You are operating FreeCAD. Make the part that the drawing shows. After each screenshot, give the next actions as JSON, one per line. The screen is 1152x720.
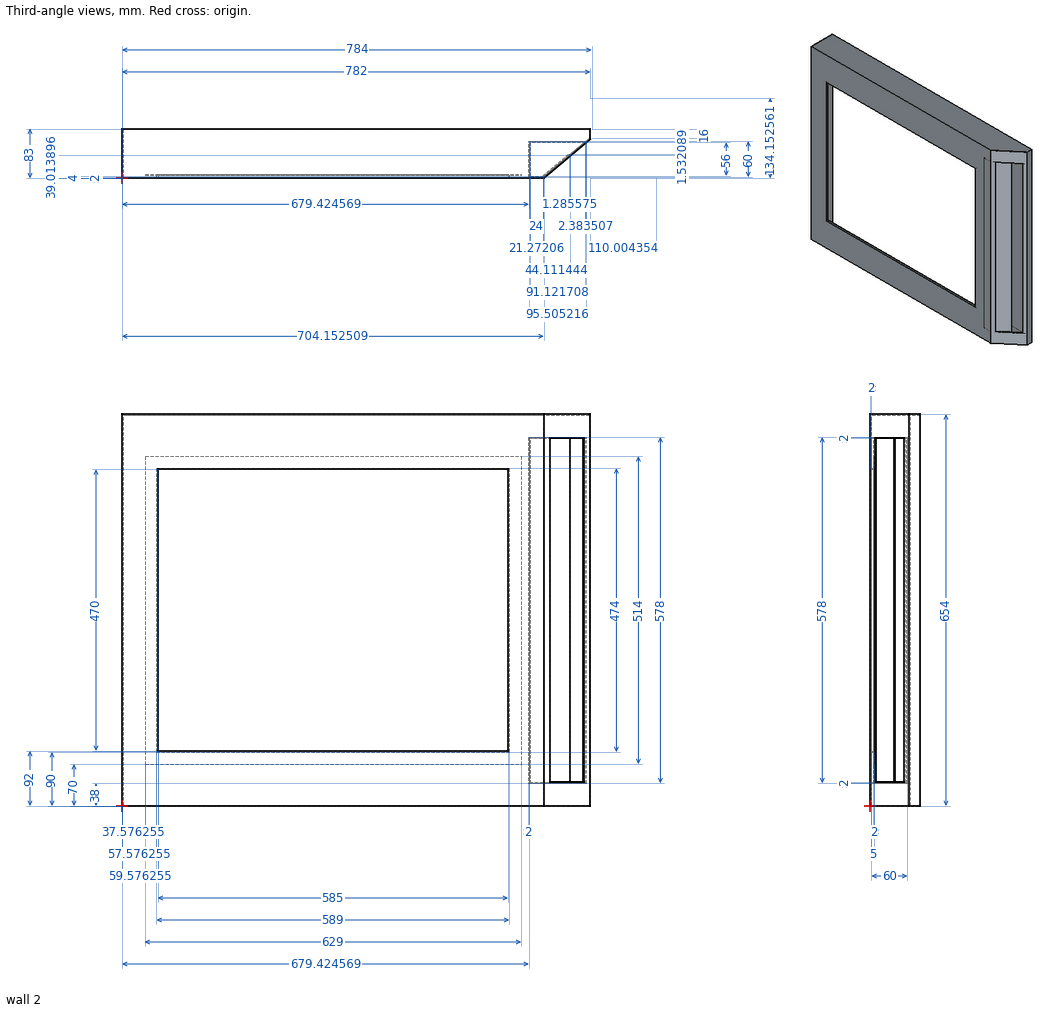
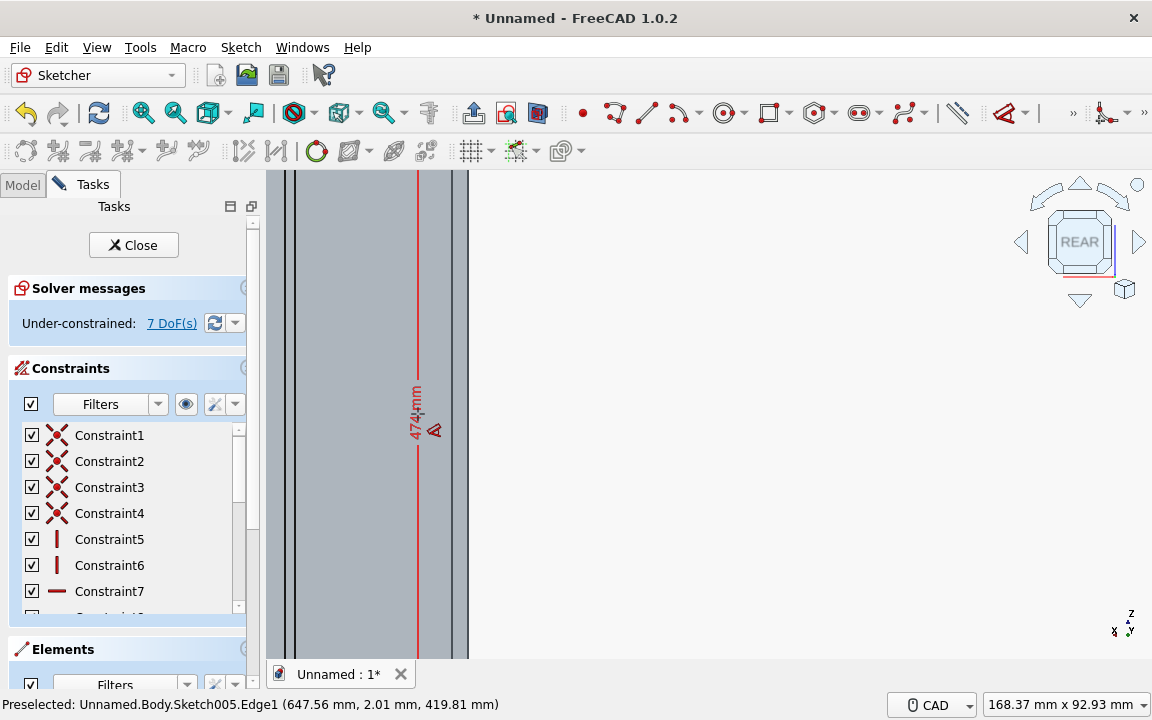
{"action": "scroll", "coordinate": [451, 334], "scroll_direction": "down", "scroll_amount": 11}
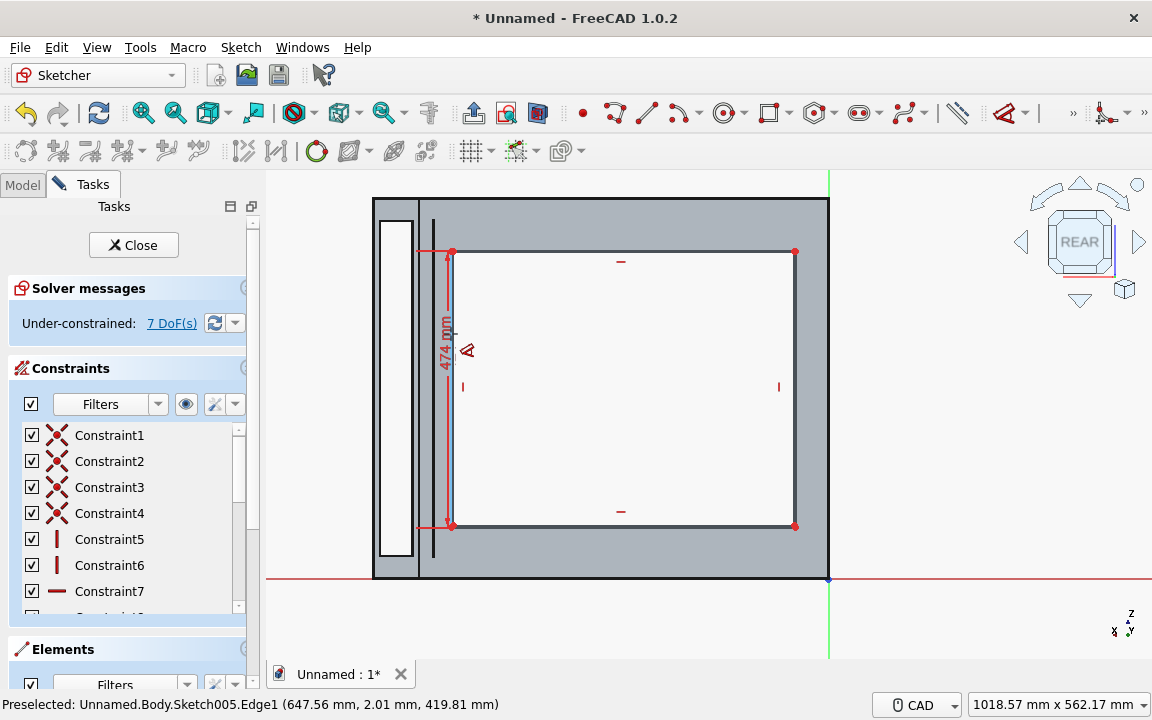
{"action": "scroll", "coordinate": [555, 528], "scroll_direction": "up", "scroll_amount": 10}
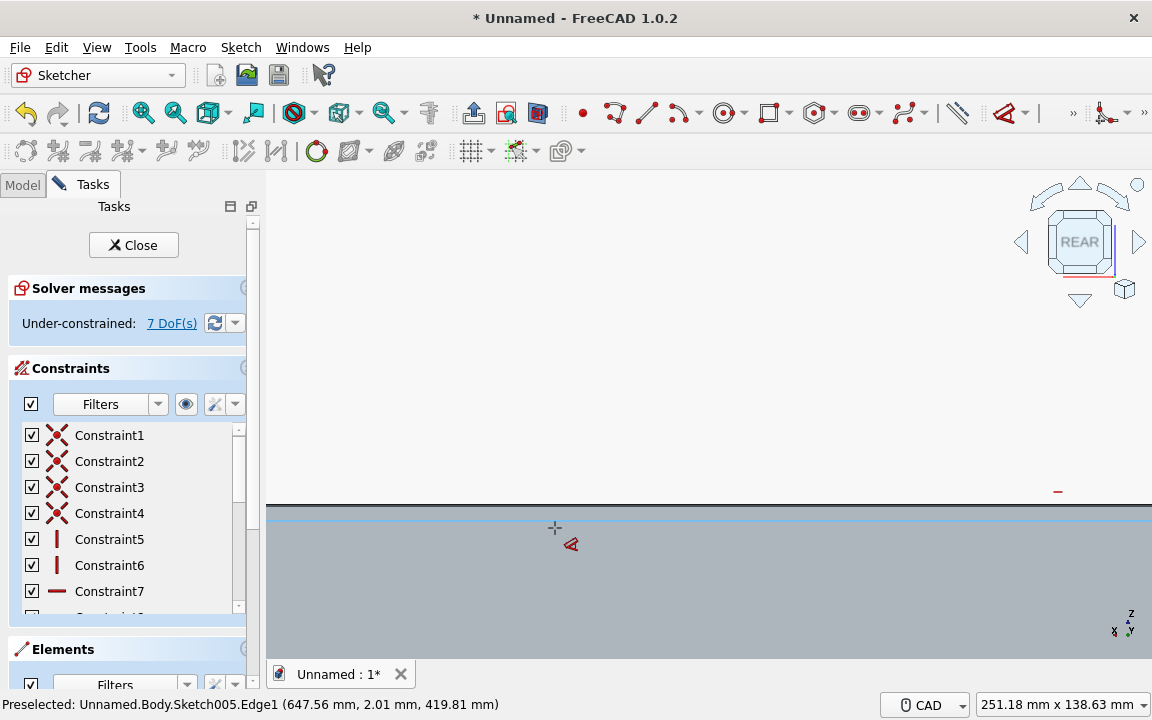
{"action": "left_click", "coordinate": [551, 521]}
{"action": "left_click", "coordinate": [640, 555]}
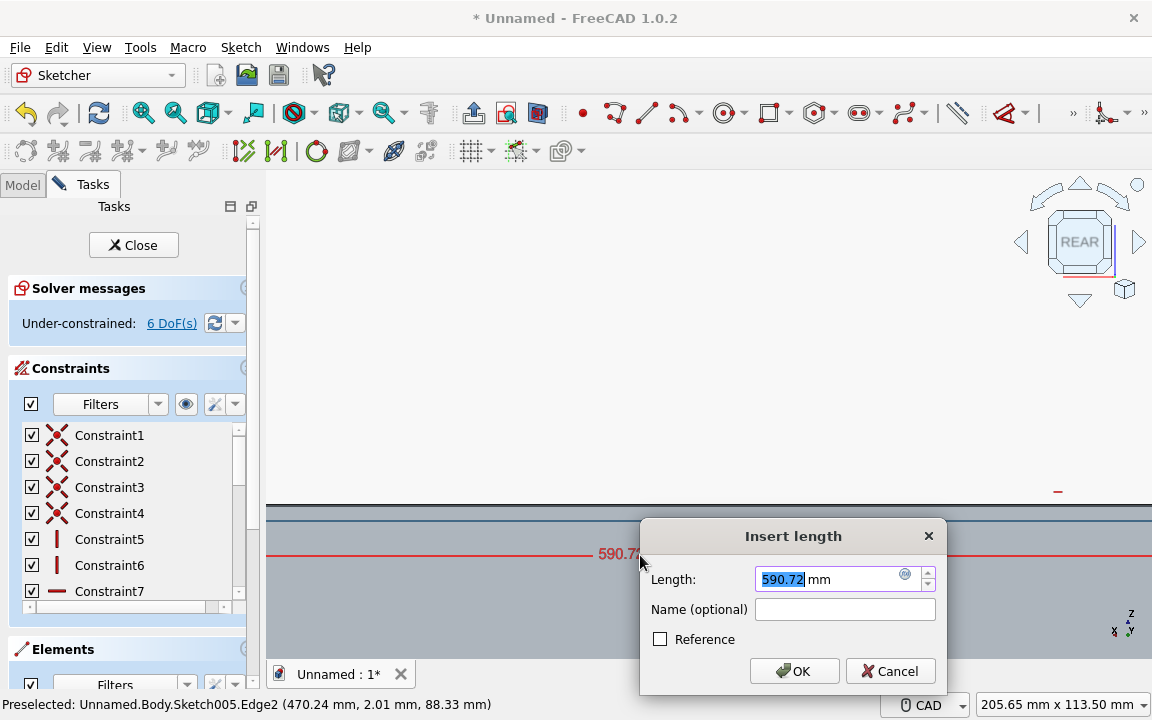
{"action": "type", "text": "589"}
{"action": "key", "text": "Return"}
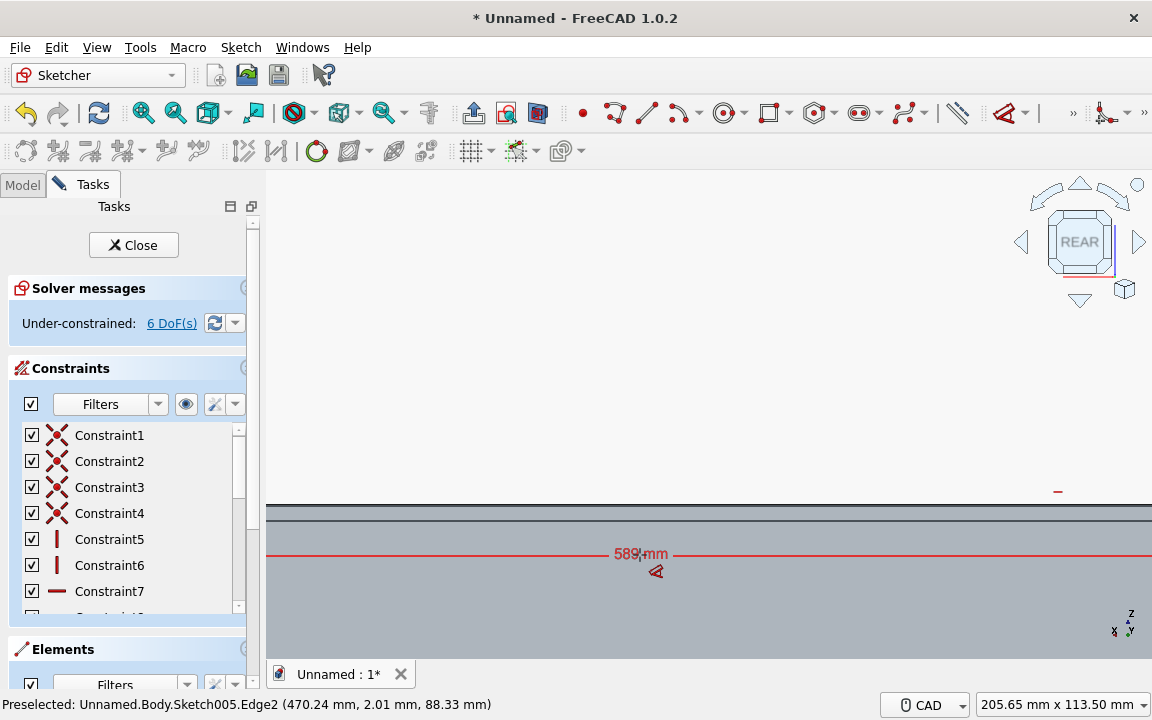
{"action": "scroll", "coordinate": [555, 528], "scroll_direction": "down", "scroll_amount": 10}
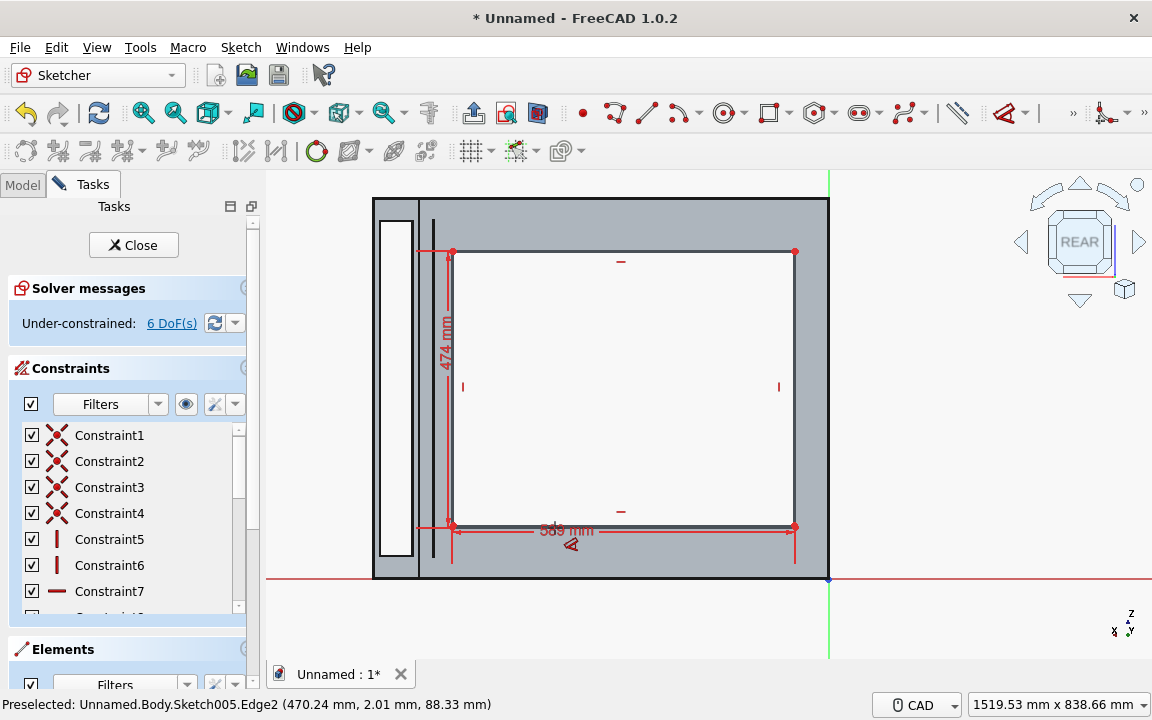
{"action": "scroll", "coordinate": [453, 334], "scroll_direction": "up", "scroll_amount": 13}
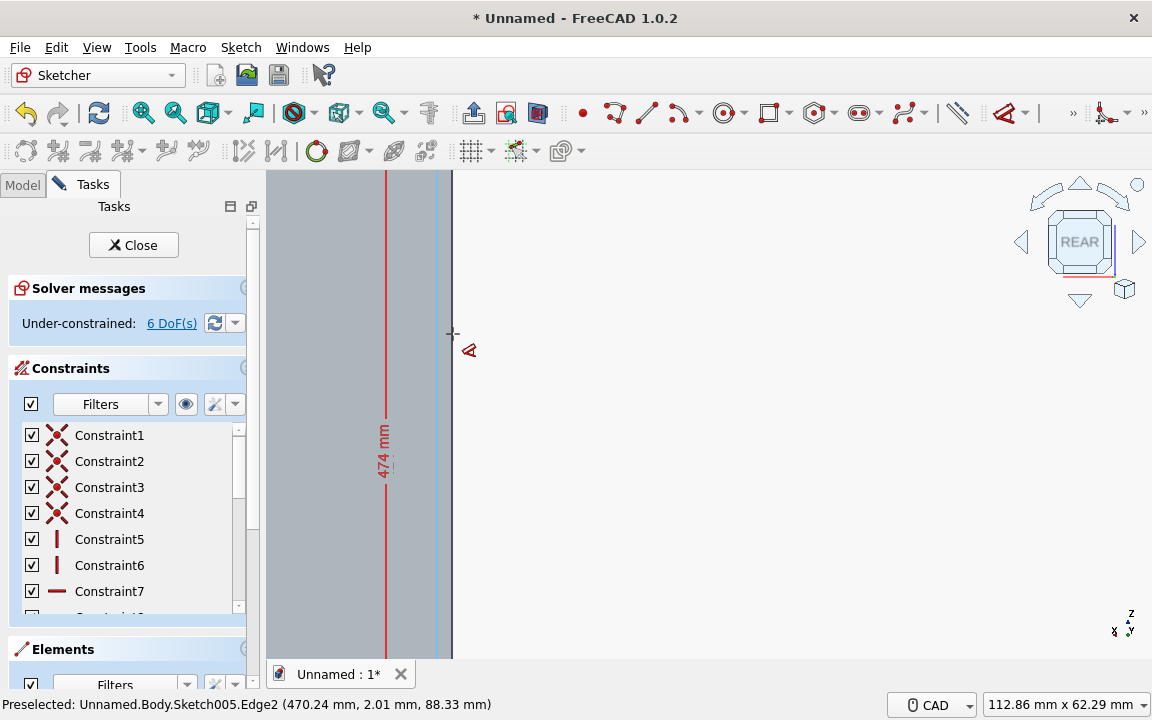
{"action": "left_click", "coordinate": [452, 327]}
{"action": "left_click", "coordinate": [418, 414]}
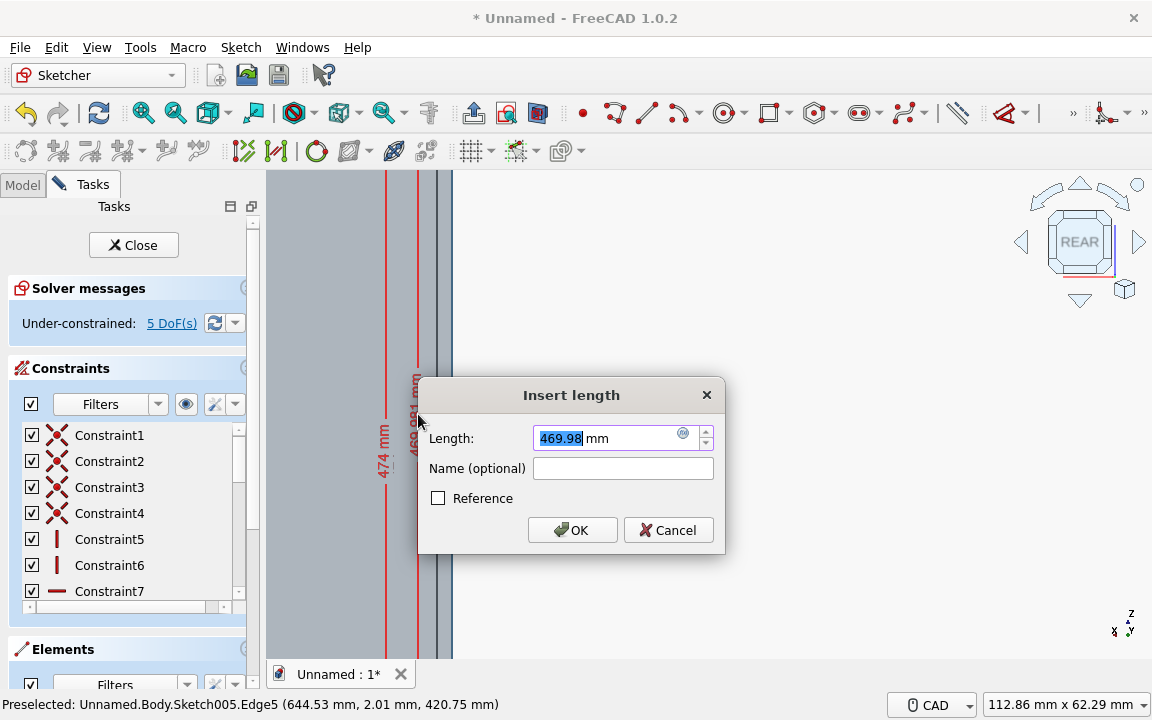
{"action": "type", "text": "470"}
{"action": "key", "text": "Return"}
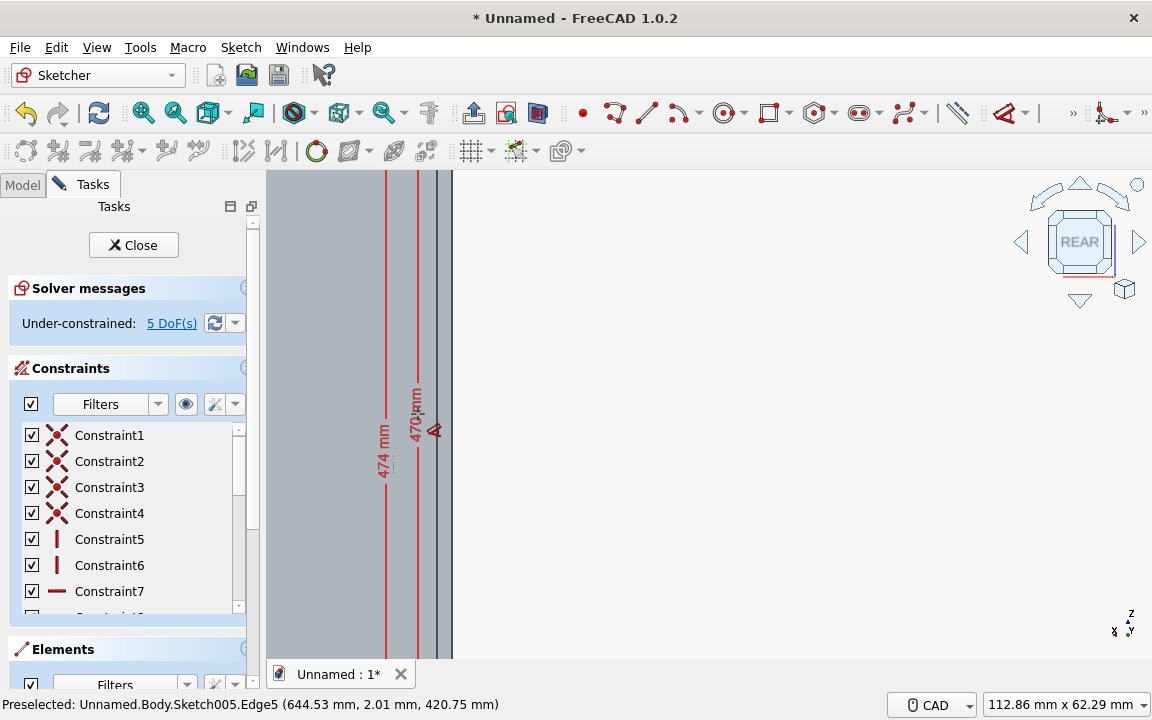
{"action": "scroll", "coordinate": [453, 334], "scroll_direction": "down", "scroll_amount": 13}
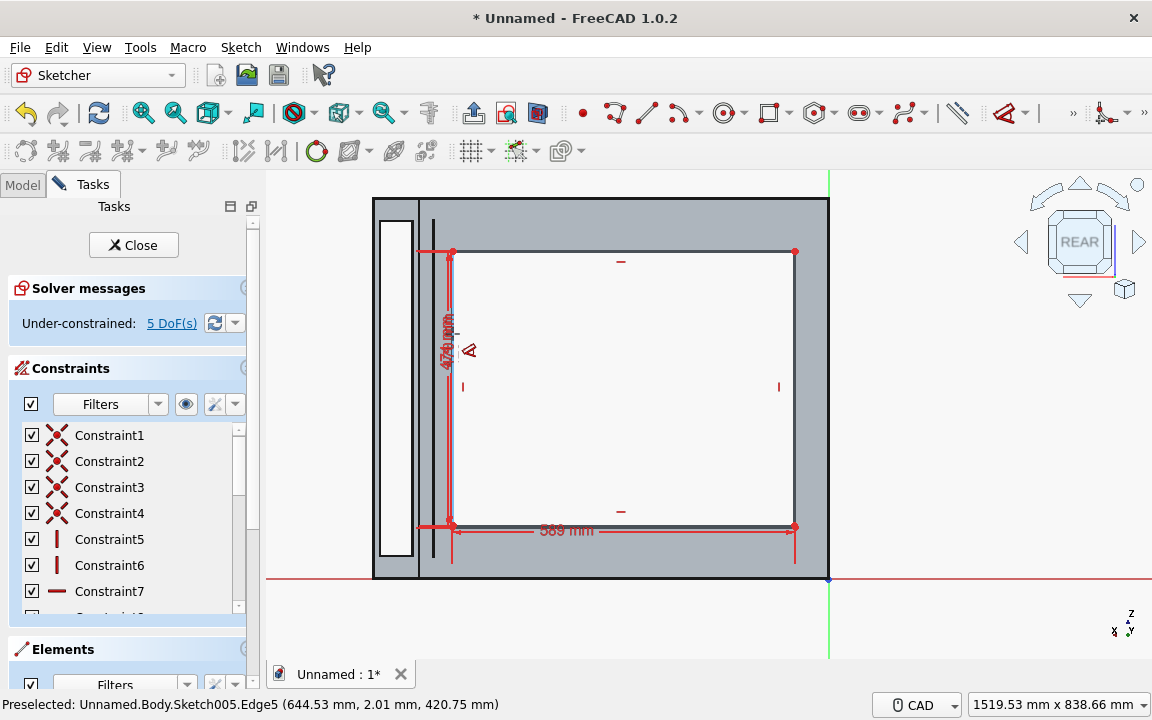
{"action": "scroll", "coordinate": [555, 526], "scroll_direction": "up", "scroll_amount": 10}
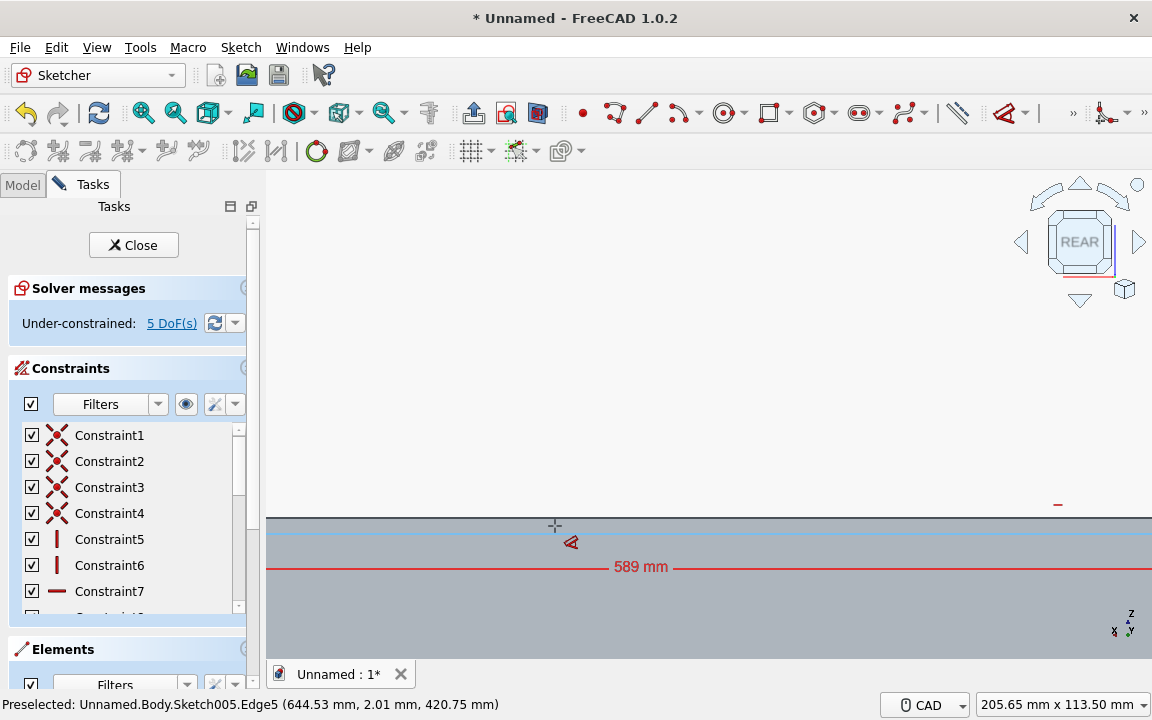
{"action": "left_click", "coordinate": [556, 518]}
{"action": "left_click", "coordinate": [481, 552]}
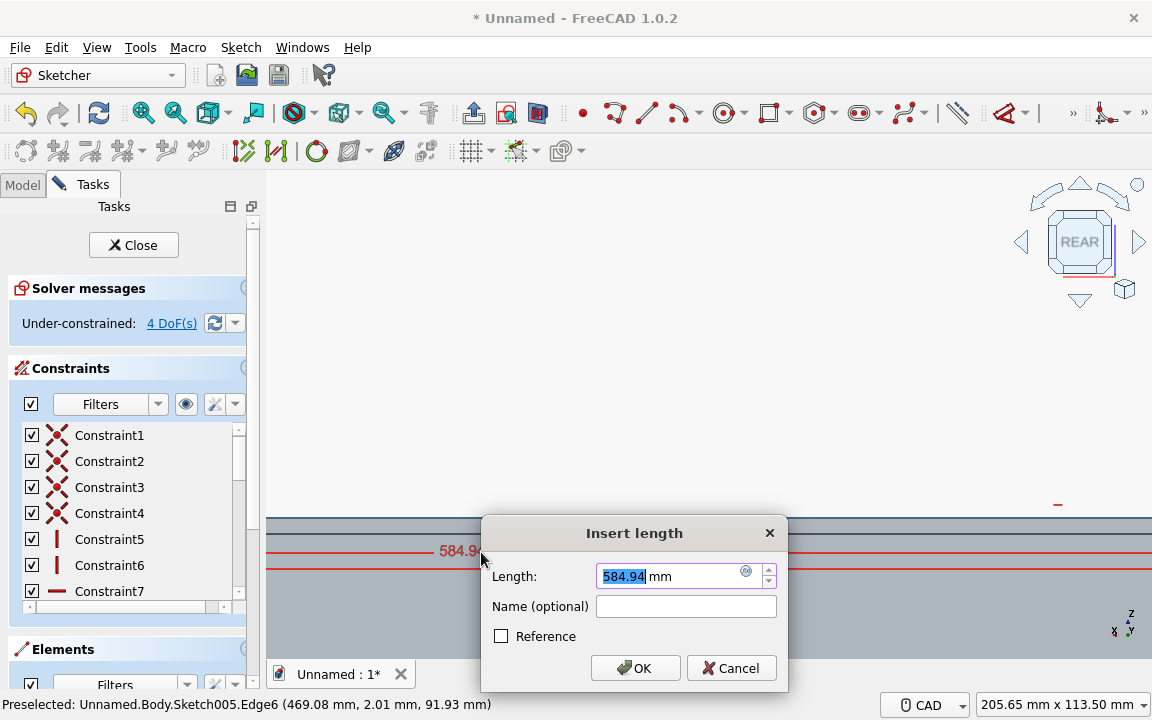
{"action": "type", "text": "585"}
{"action": "key", "text": "Return"}